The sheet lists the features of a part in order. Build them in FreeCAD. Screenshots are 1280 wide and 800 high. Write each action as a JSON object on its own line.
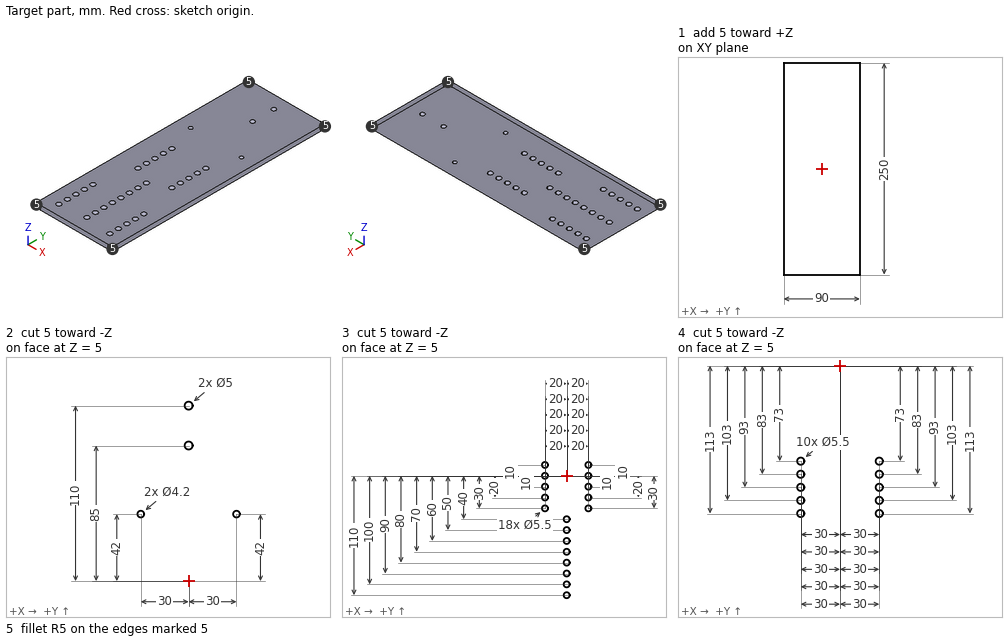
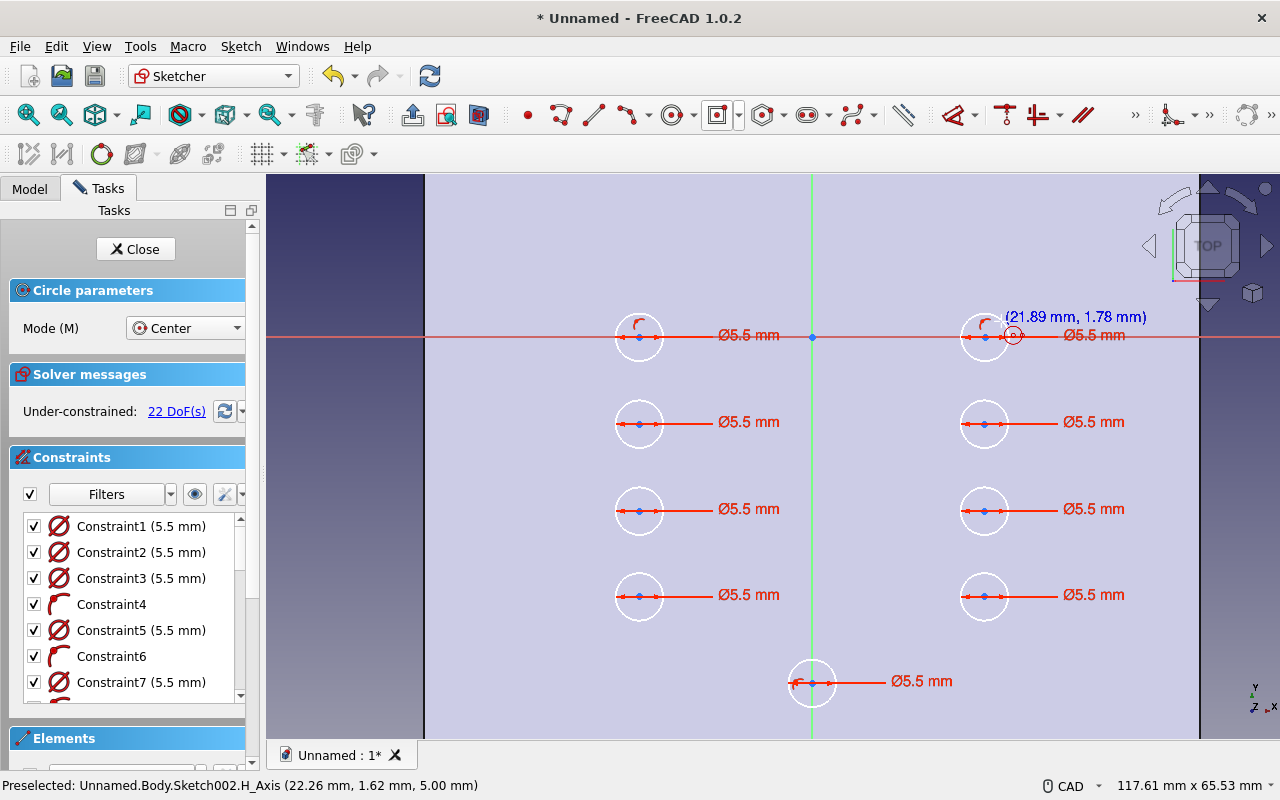
{"action": "left_click", "coordinate": [640, 251]}
{"action": "mouse_move", "coordinate": [657, 234]}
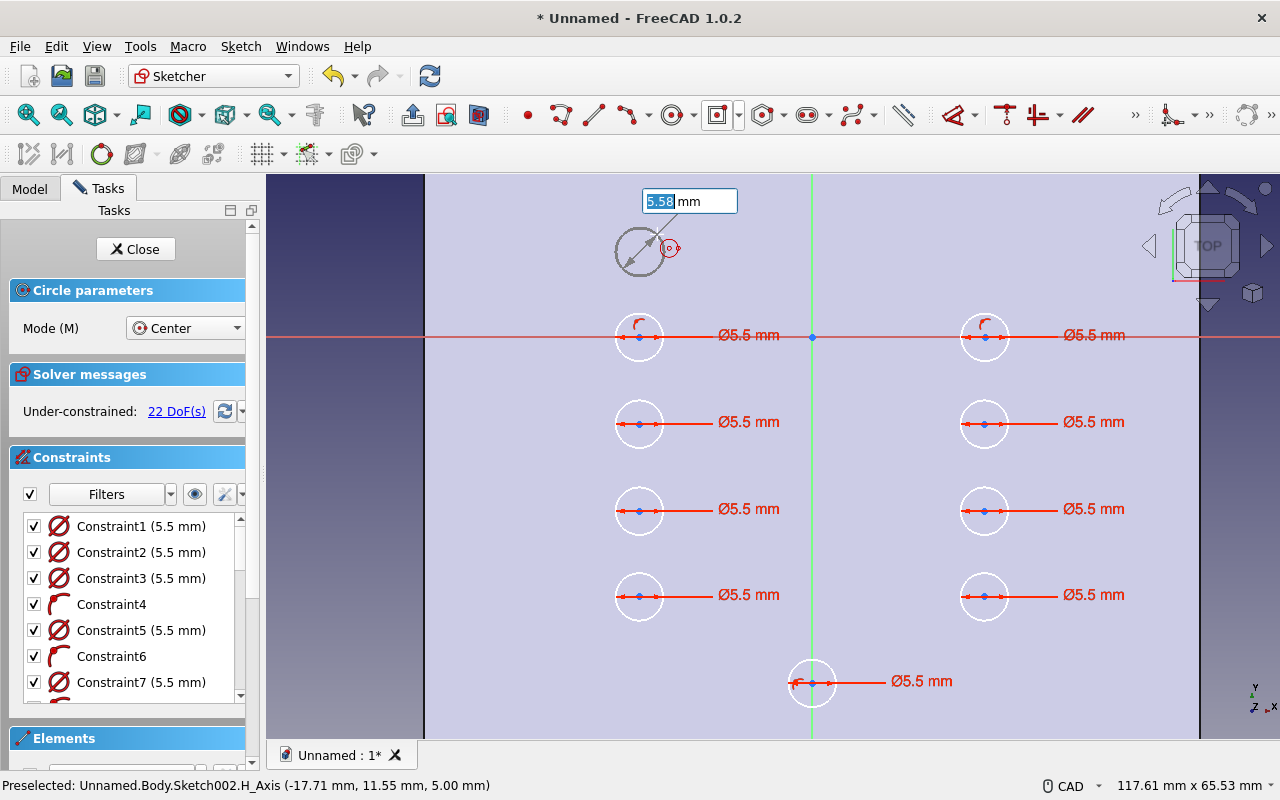
{"action": "type", "text": "5.5"}
{"action": "key", "text": "Return"}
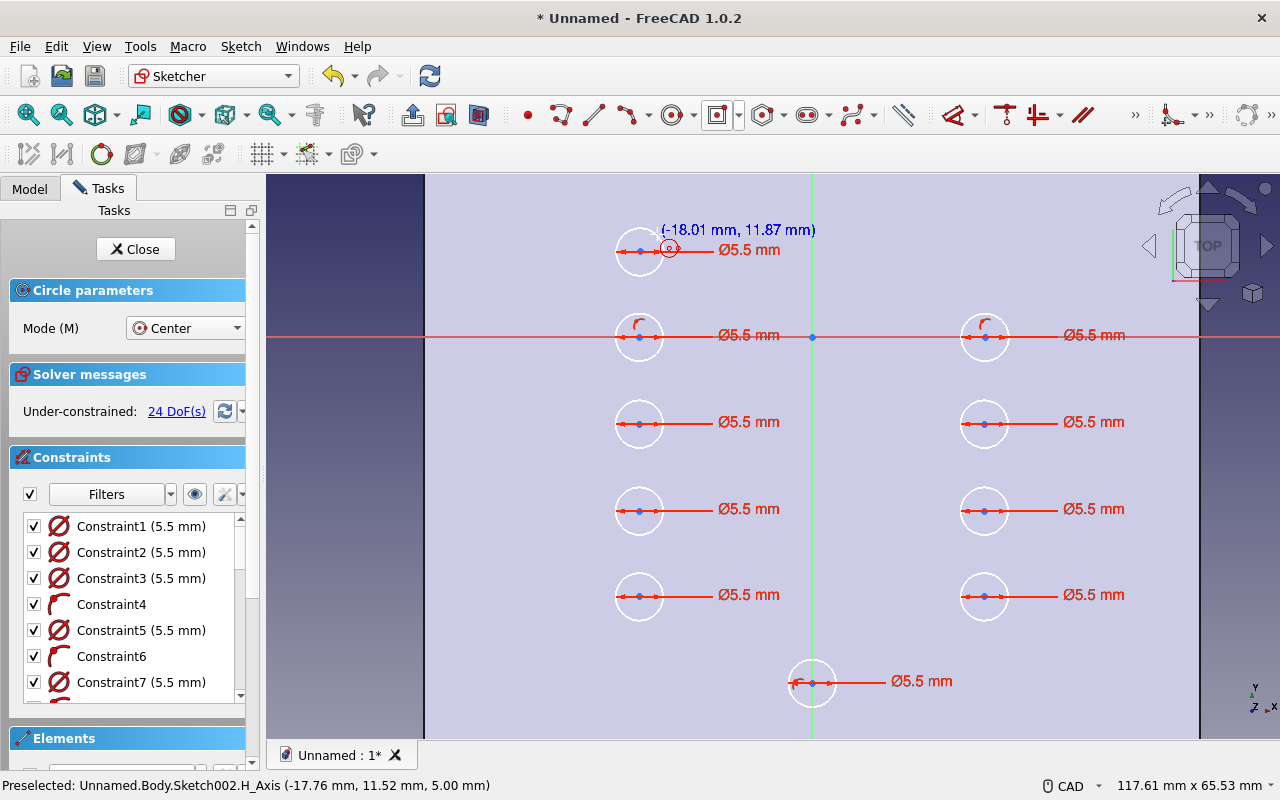
{"action": "left_click", "coordinate": [985, 251]}
{"action": "mouse_move", "coordinate": [1001, 234]}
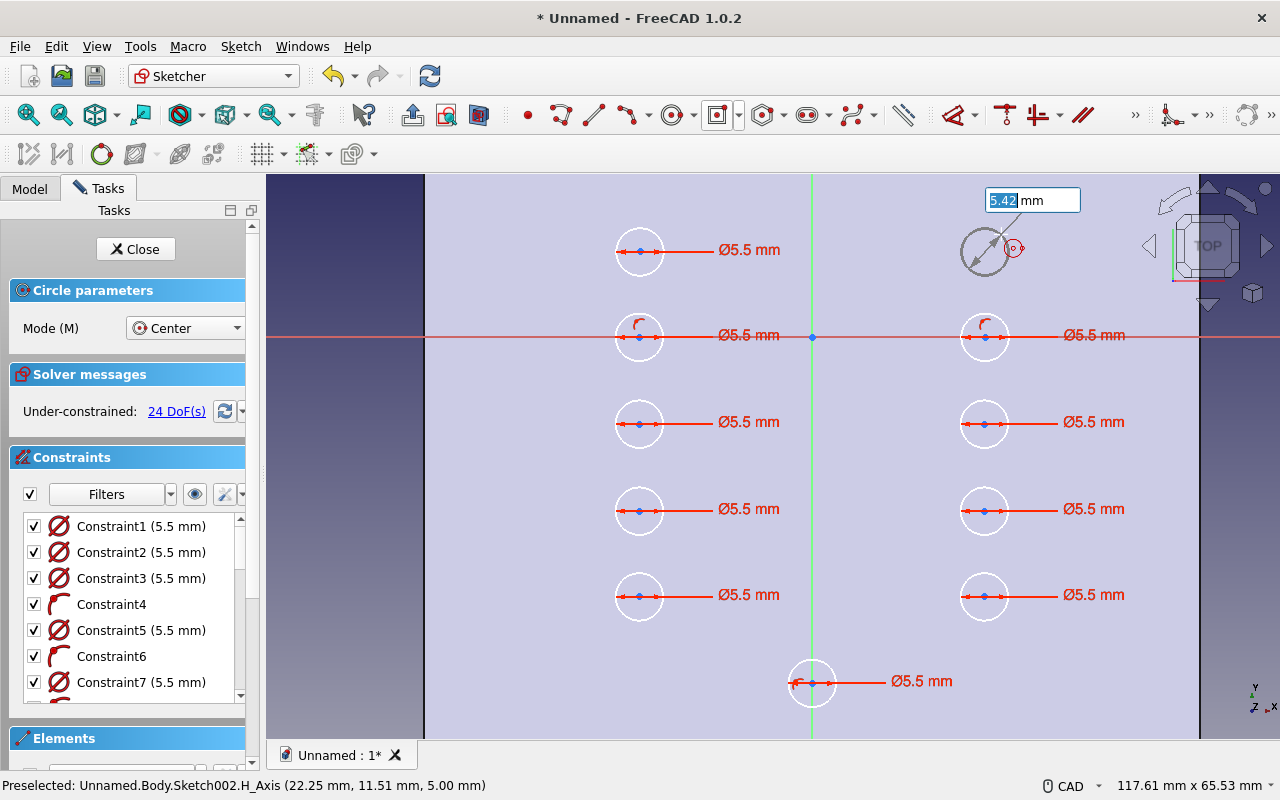
{"action": "type", "text": "5.5"}
{"action": "key", "text": "Return"}
{"action": "key", "text": "Escape"}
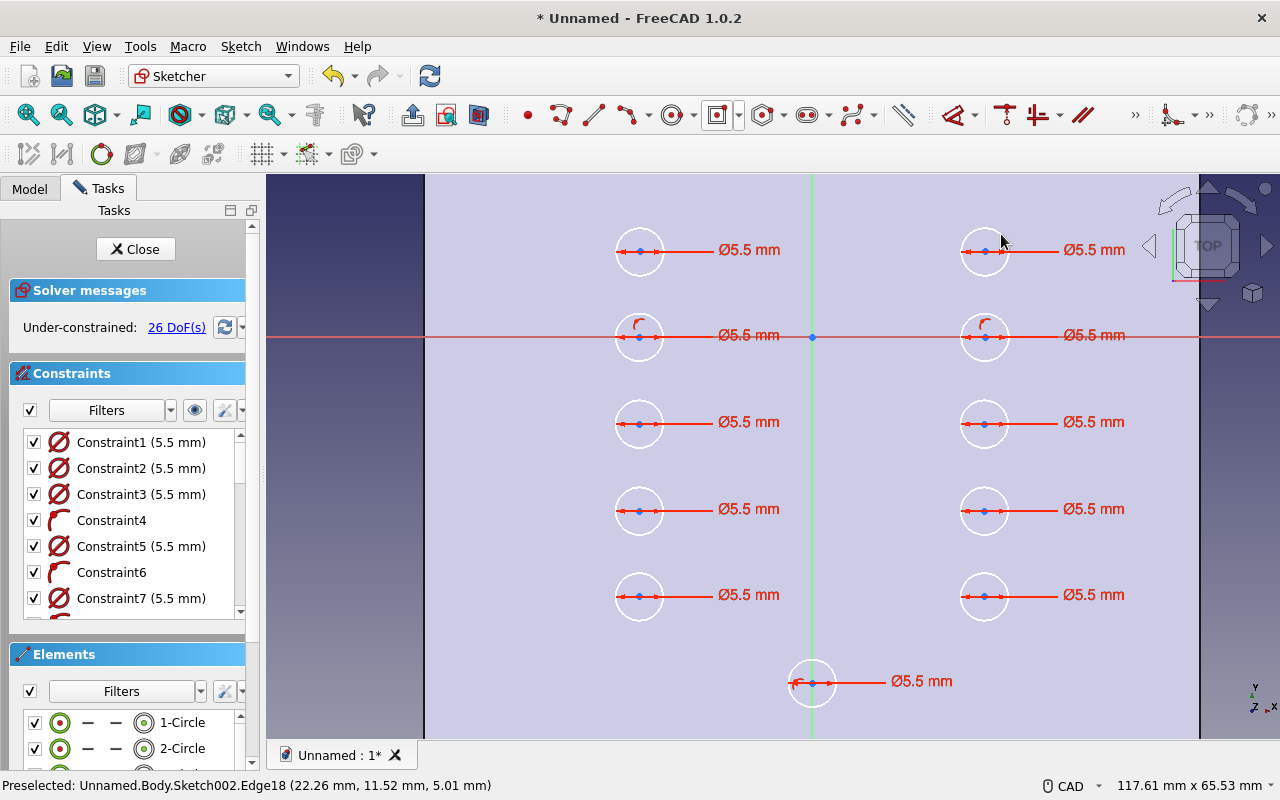
{"action": "key", "text": "d"}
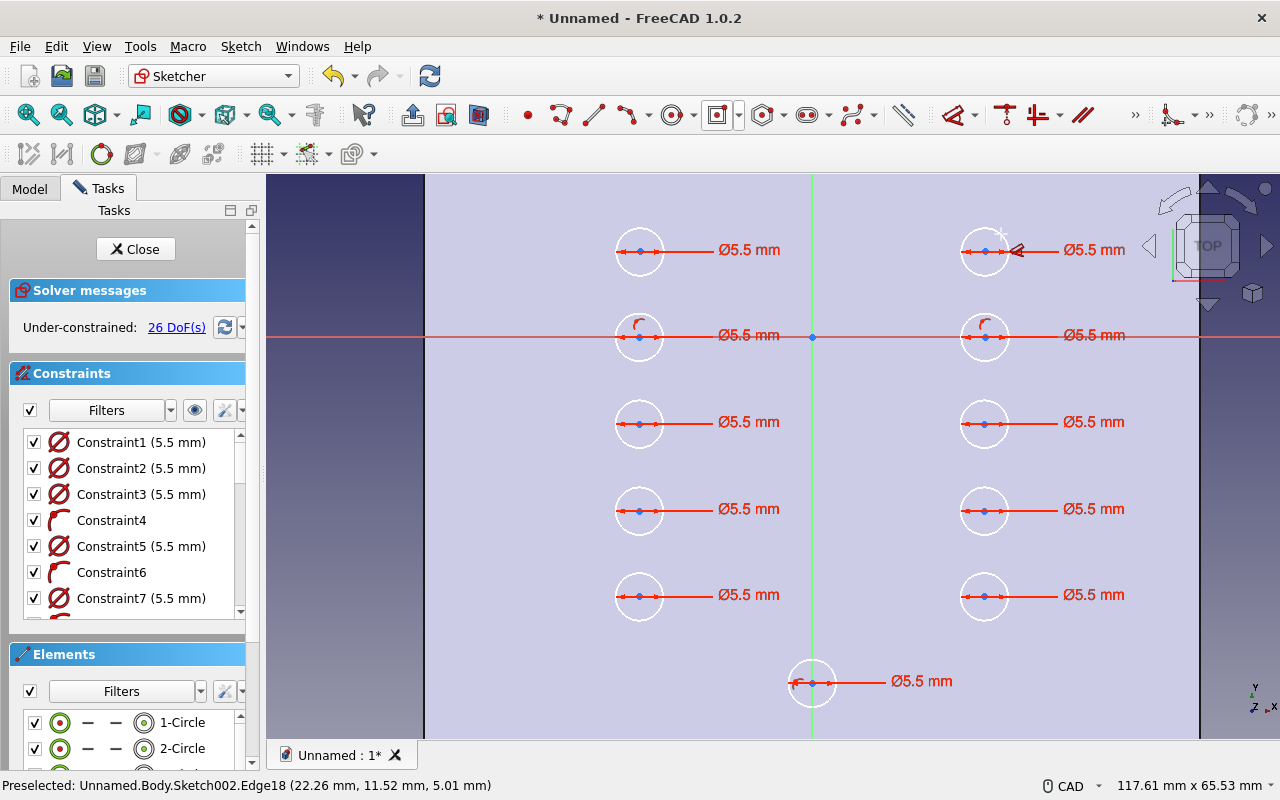
{"action": "left_click", "coordinate": [639, 597]}
{"action": "left_click", "coordinate": [726, 303]}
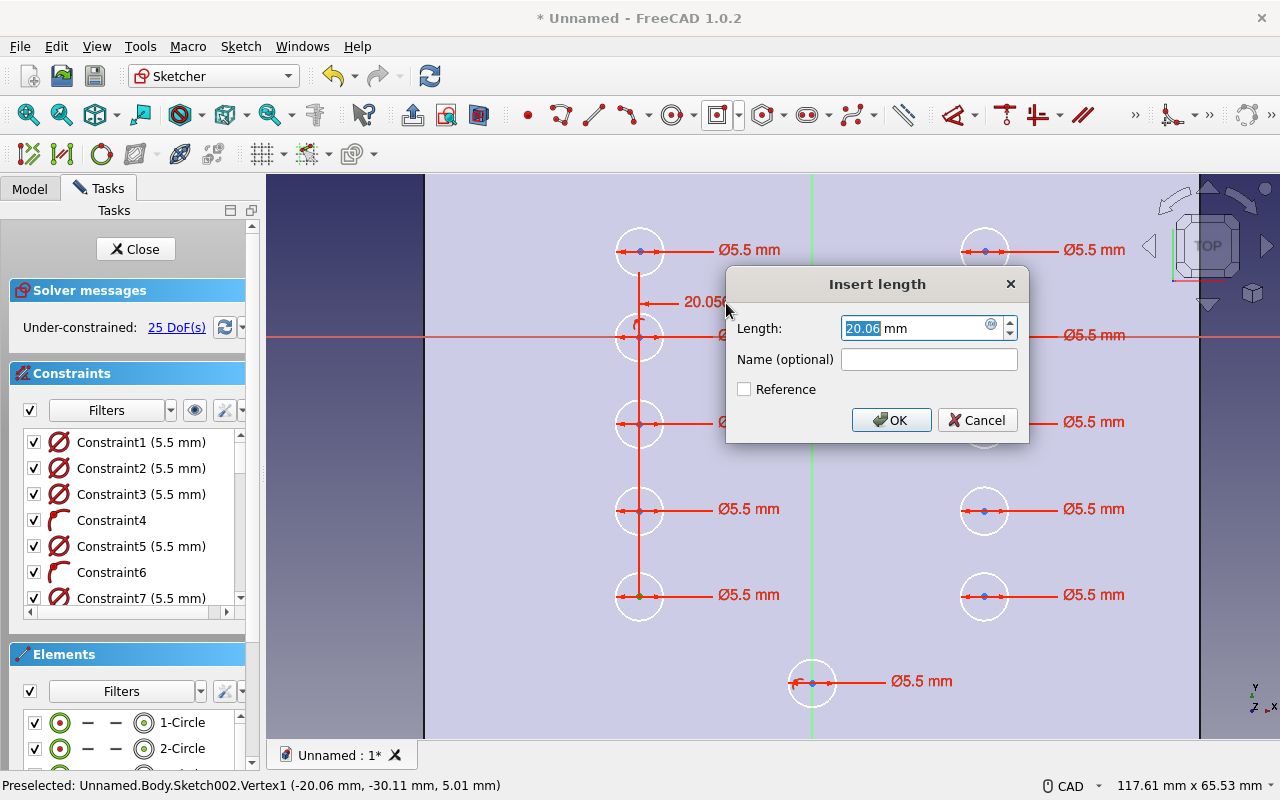
{"action": "type", "text": "20"}
{"action": "key", "text": "Return"}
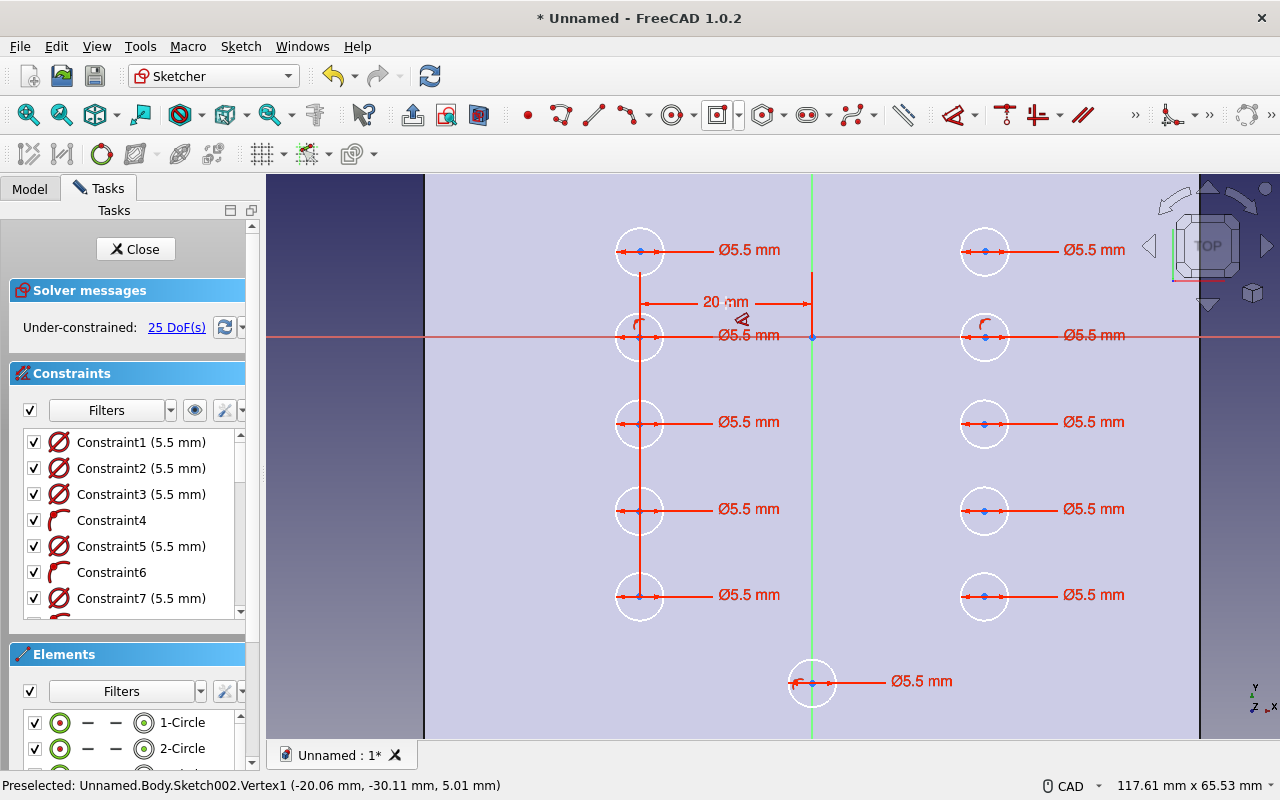
{"action": "left_click", "coordinate": [640, 597]}
{"action": "left_click", "coordinate": [606, 467]}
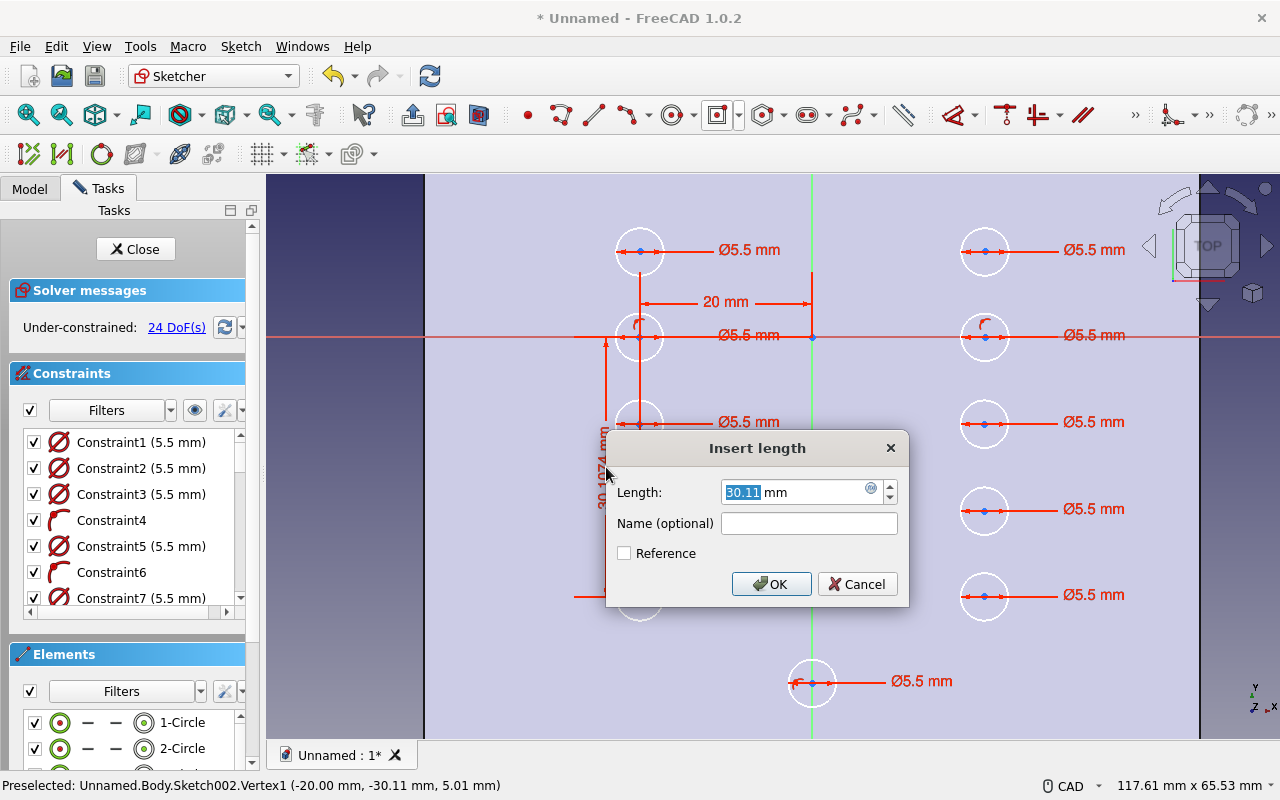
{"action": "type", "text": "30"}
{"action": "key", "text": "Return"}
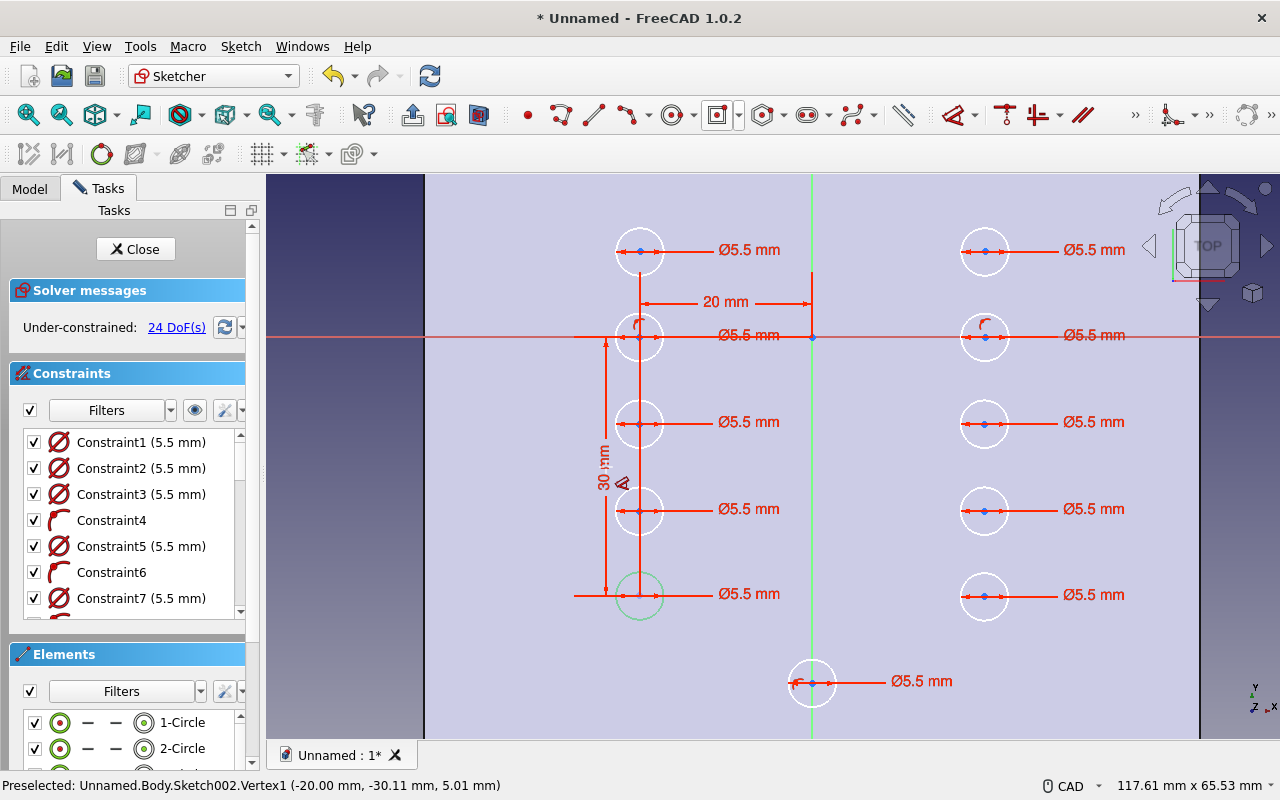
{"action": "left_click", "coordinate": [984, 597]}
{"action": "left_click", "coordinate": [898, 303]}